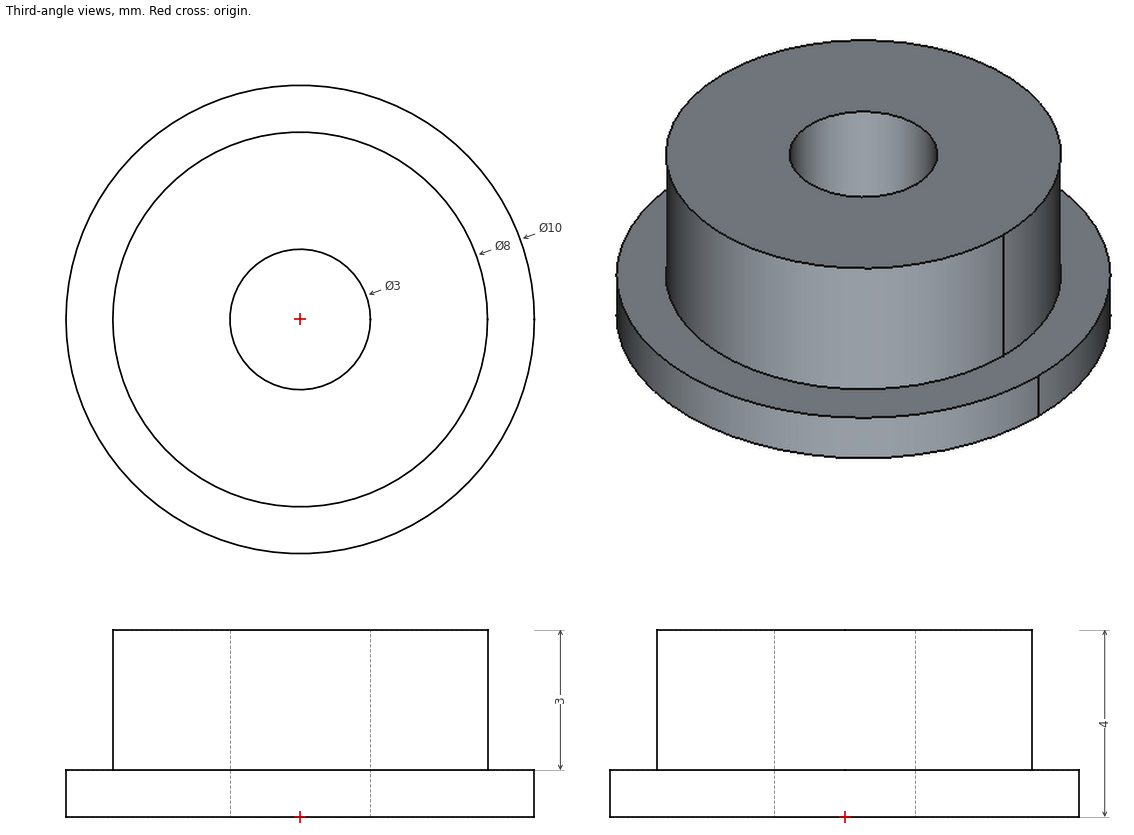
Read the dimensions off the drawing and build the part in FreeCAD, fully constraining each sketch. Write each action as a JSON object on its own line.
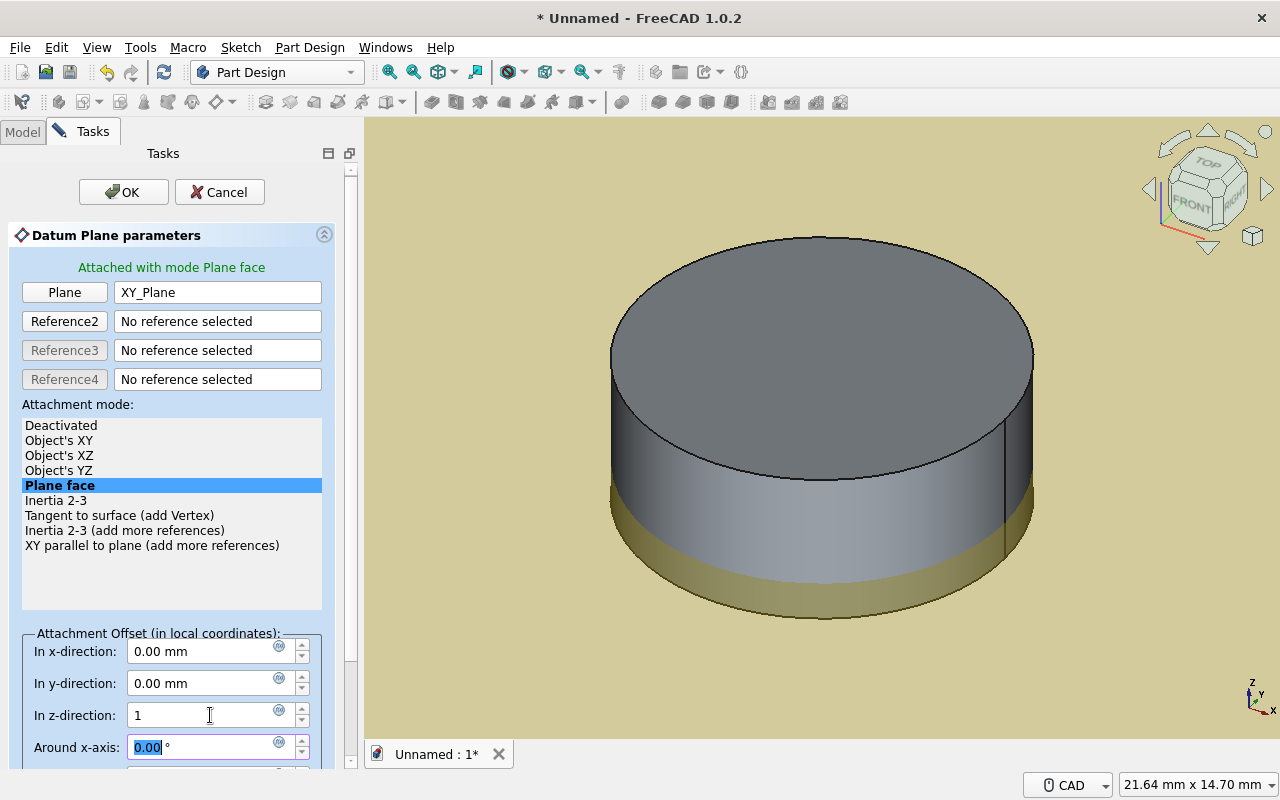
{"action": "left_click", "coordinate": [124, 192]}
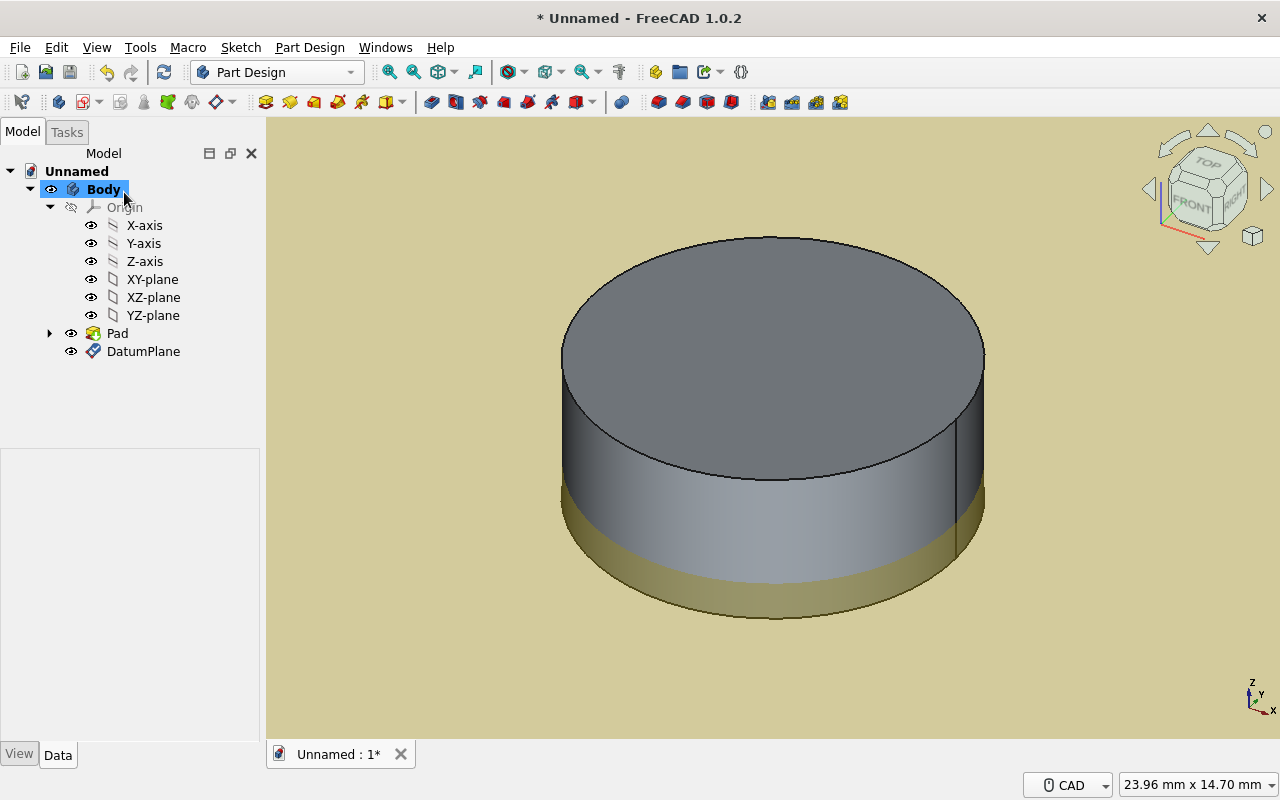
{"action": "left_click", "coordinate": [116, 351]}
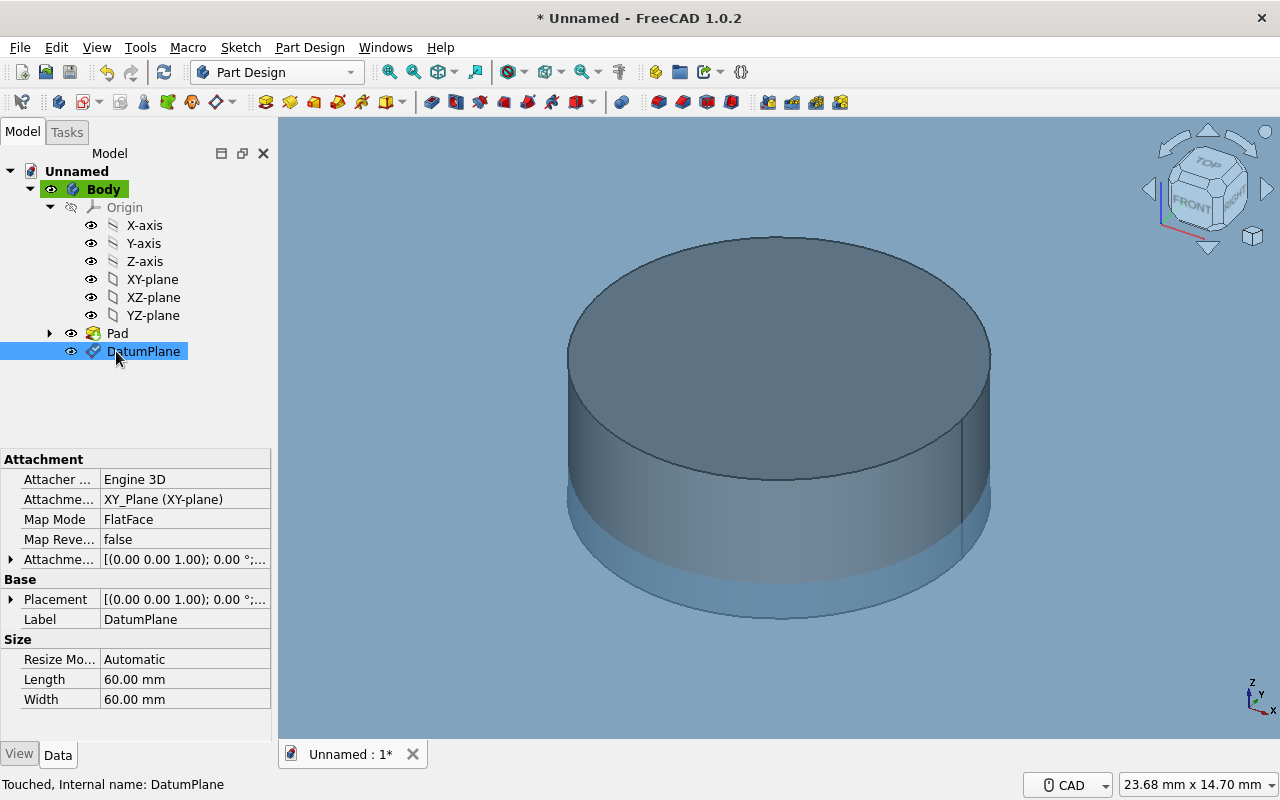
{"action": "left_click", "coordinate": [84, 102]}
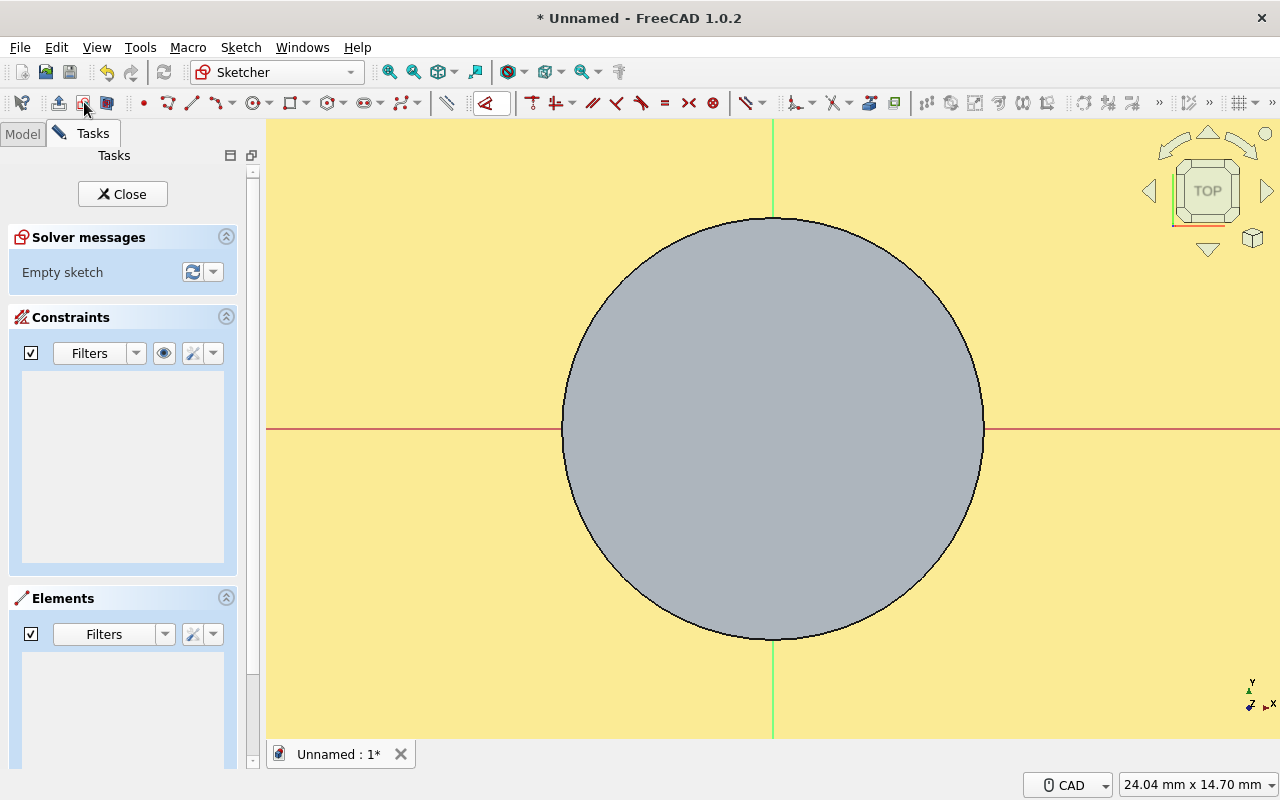
{"action": "left_click", "coordinate": [108, 104]}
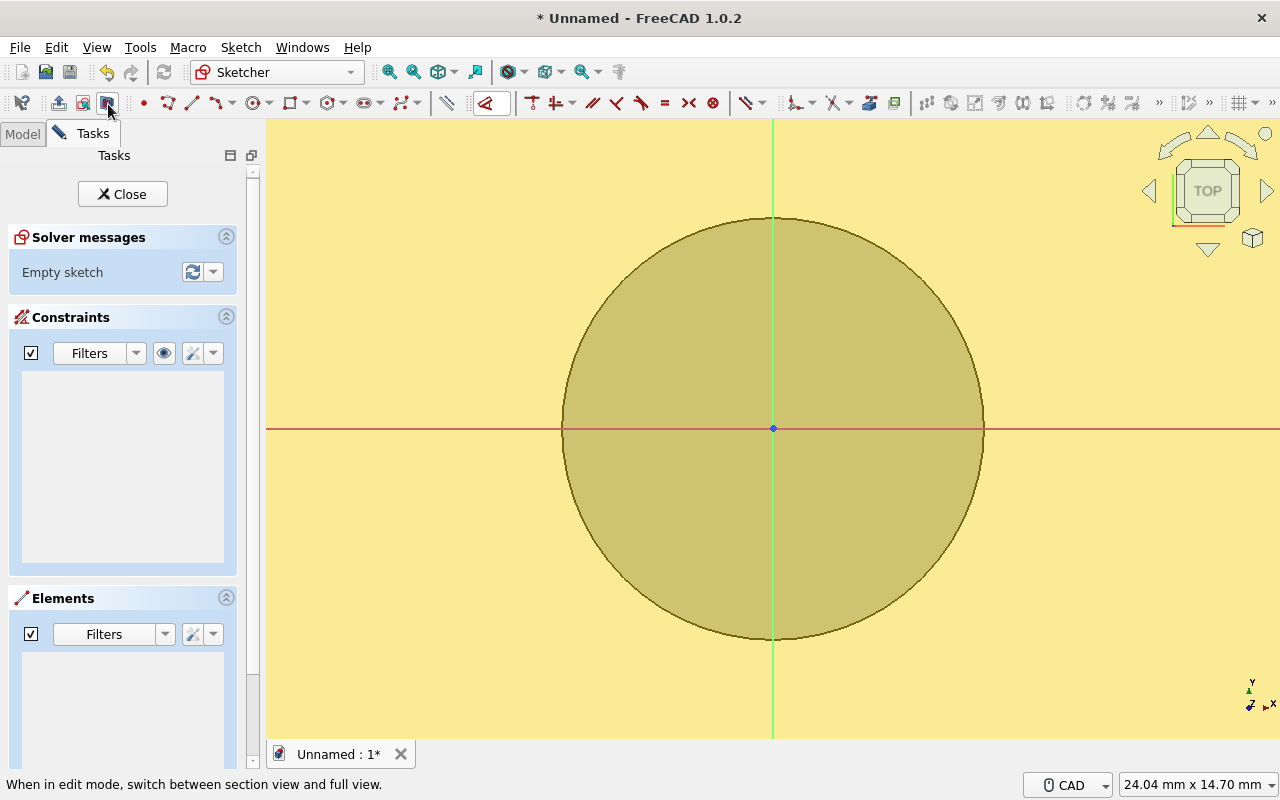
{"action": "left_click", "coordinate": [254, 104]}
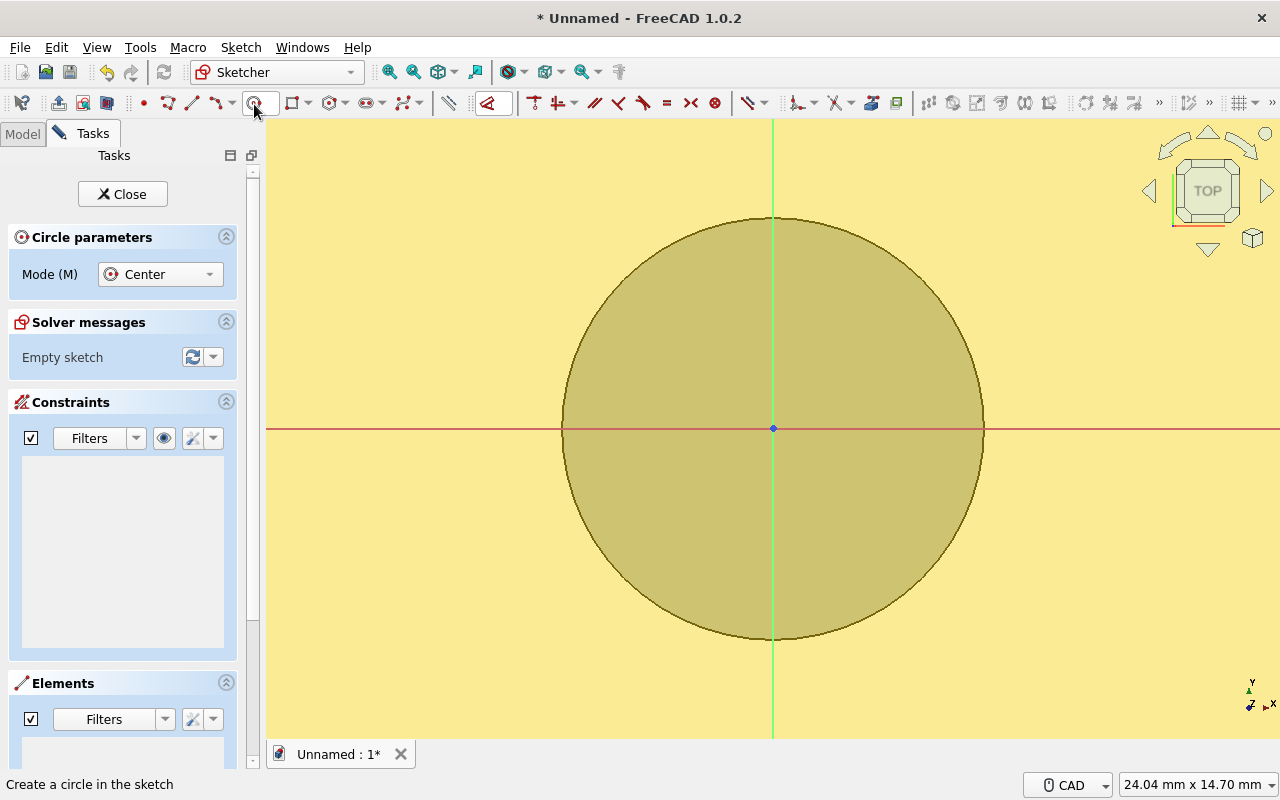
{"action": "left_click", "coordinate": [773, 429]}
{"action": "left_click", "coordinate": [922, 280]}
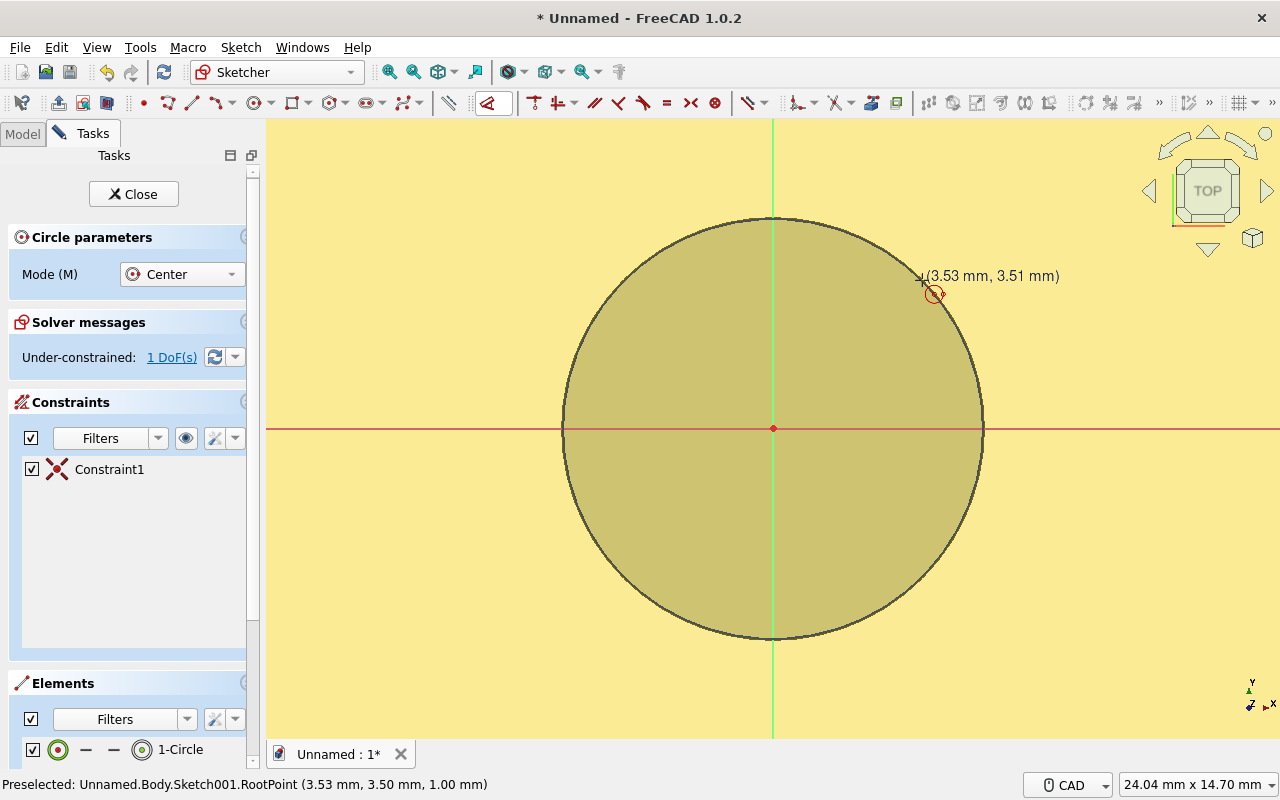
{"action": "left_click", "coordinate": [773, 429]}
{"action": "left_click", "coordinate": [892, 310]}
{"action": "key", "text": "Escape"}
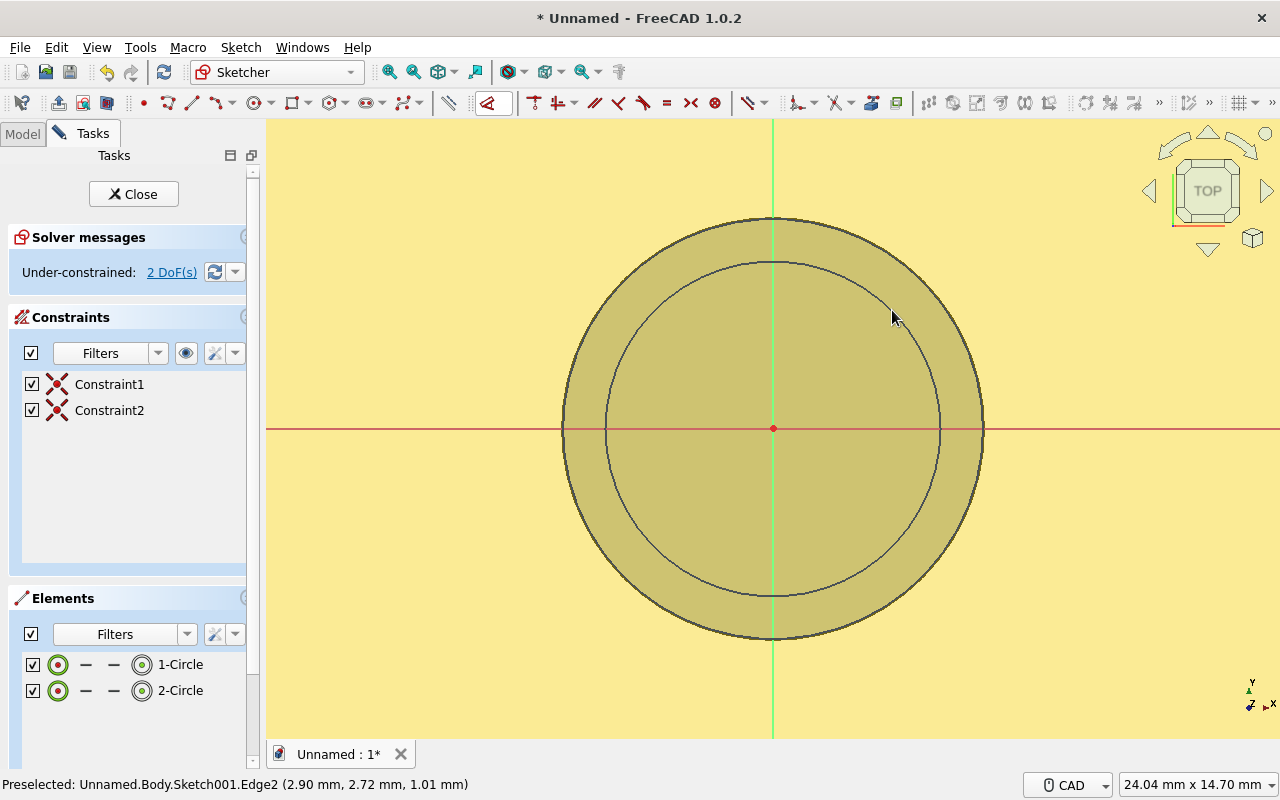
{"action": "left_click", "coordinate": [921, 280]}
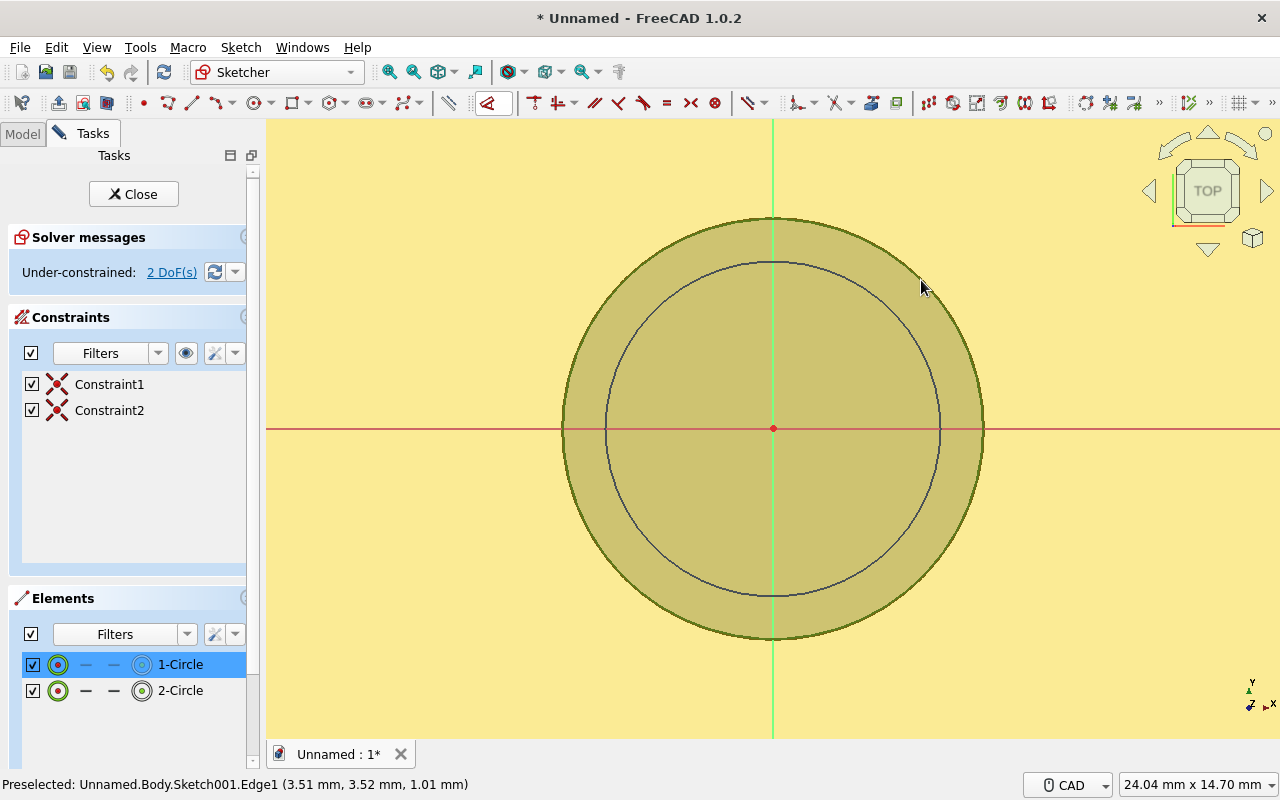
{"action": "key", "text": "k o"}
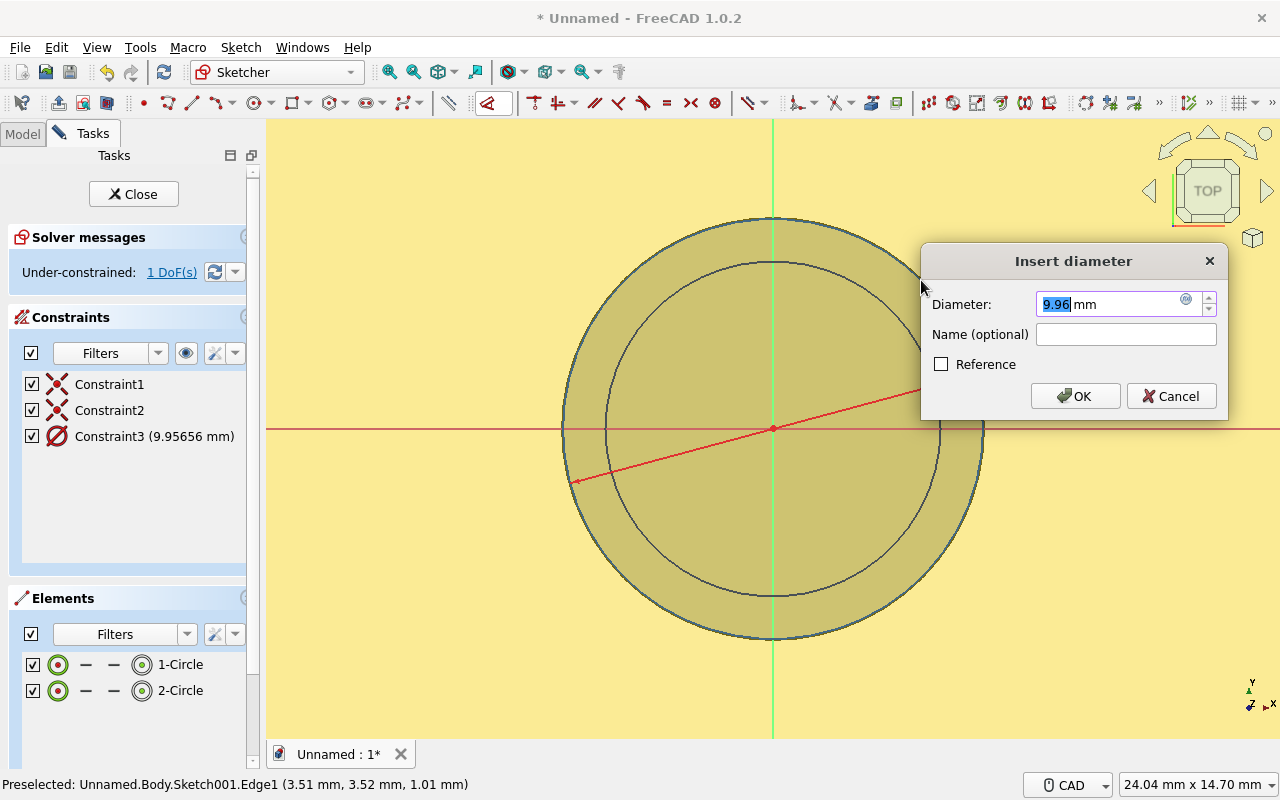
{"action": "type", "text": "10"}
{"action": "key", "text": "Return"}